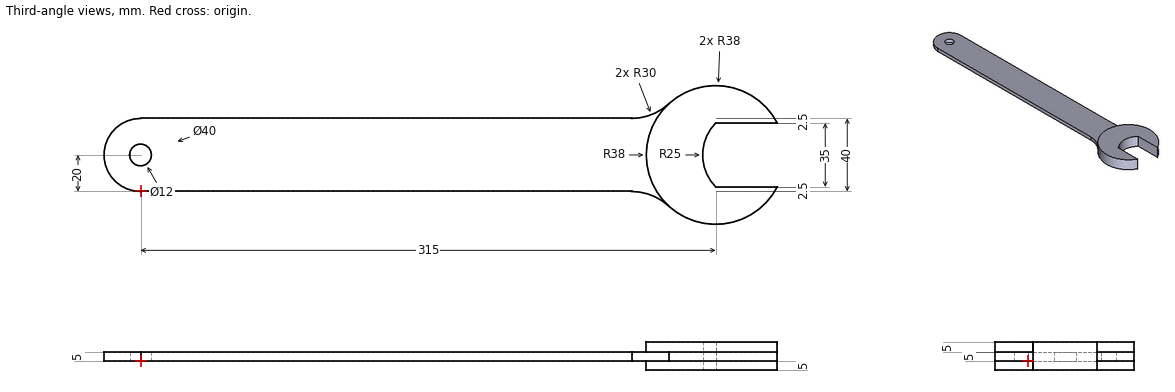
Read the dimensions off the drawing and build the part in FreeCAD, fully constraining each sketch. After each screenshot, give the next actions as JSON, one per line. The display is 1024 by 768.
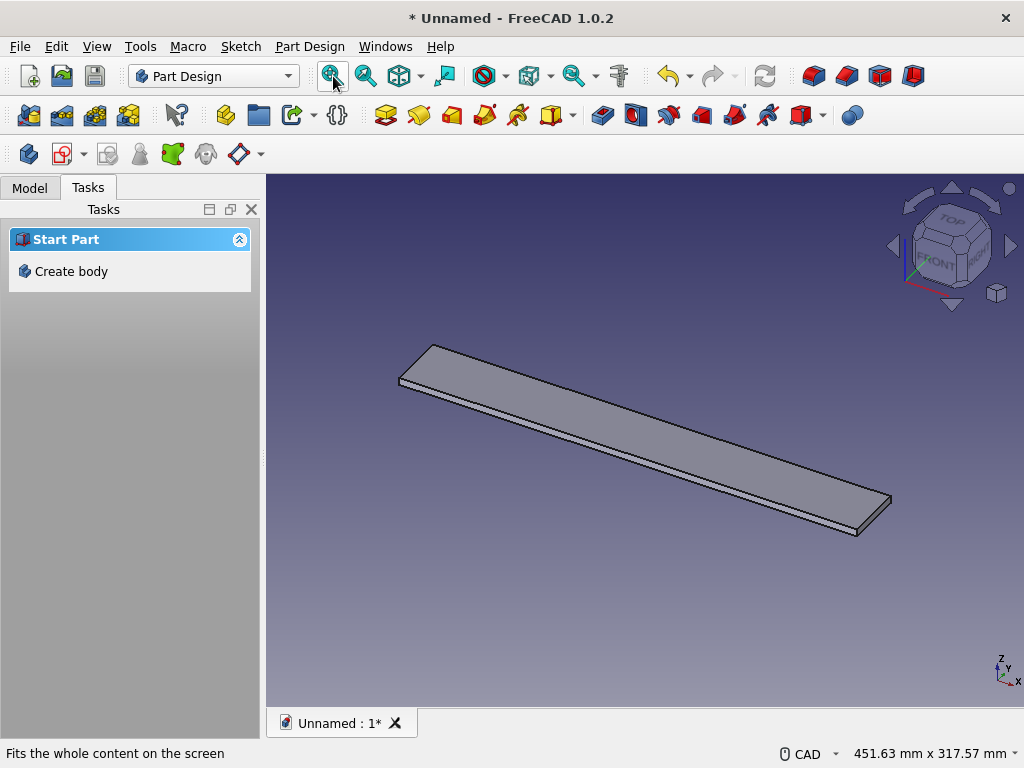
{"action": "left_click", "coordinate": [841, 501]}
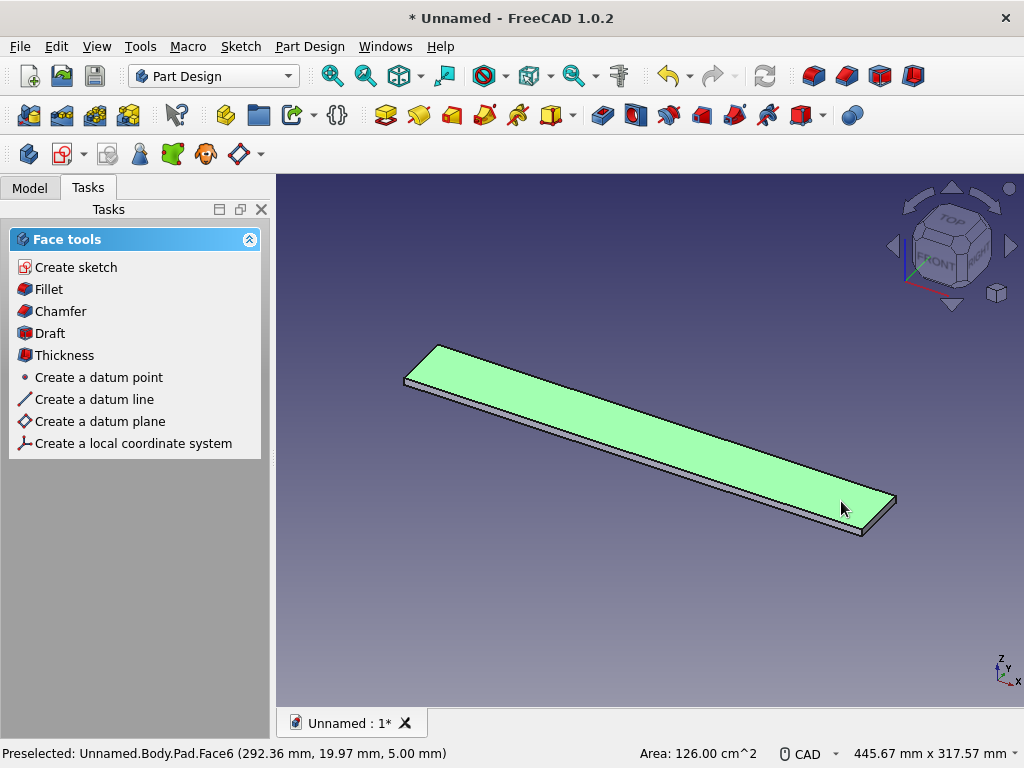
{"action": "left_click", "coordinate": [62, 154]}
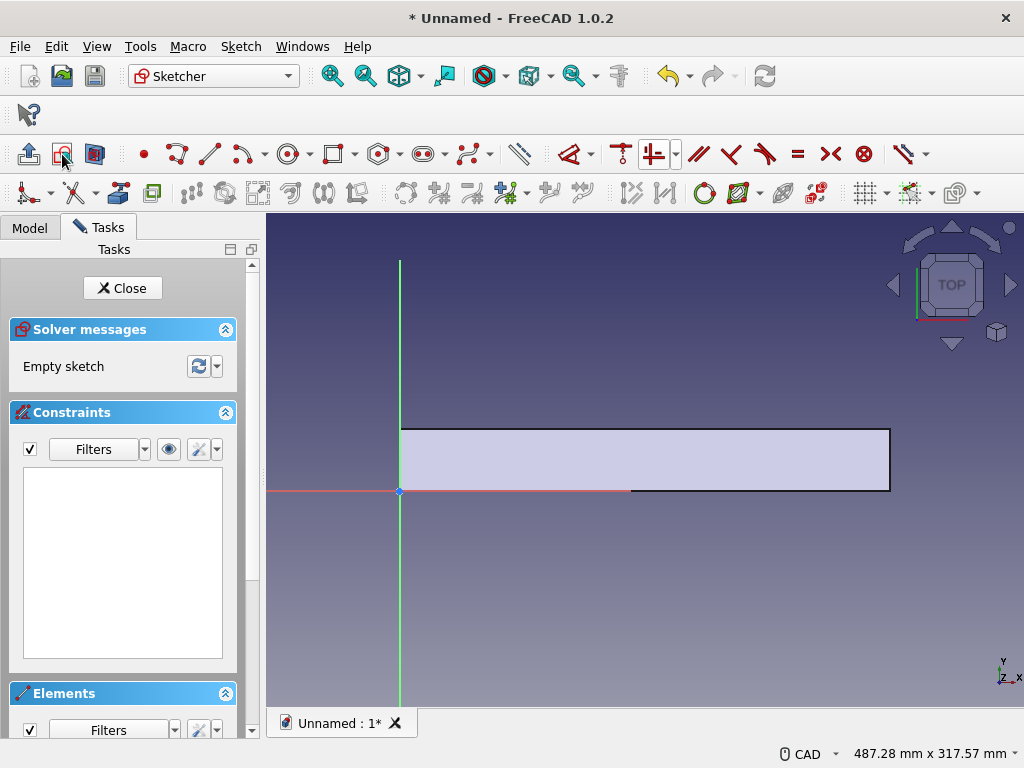
{"action": "scroll", "coordinate": [355, 460], "scroll_direction": "up", "scroll_amount": 8}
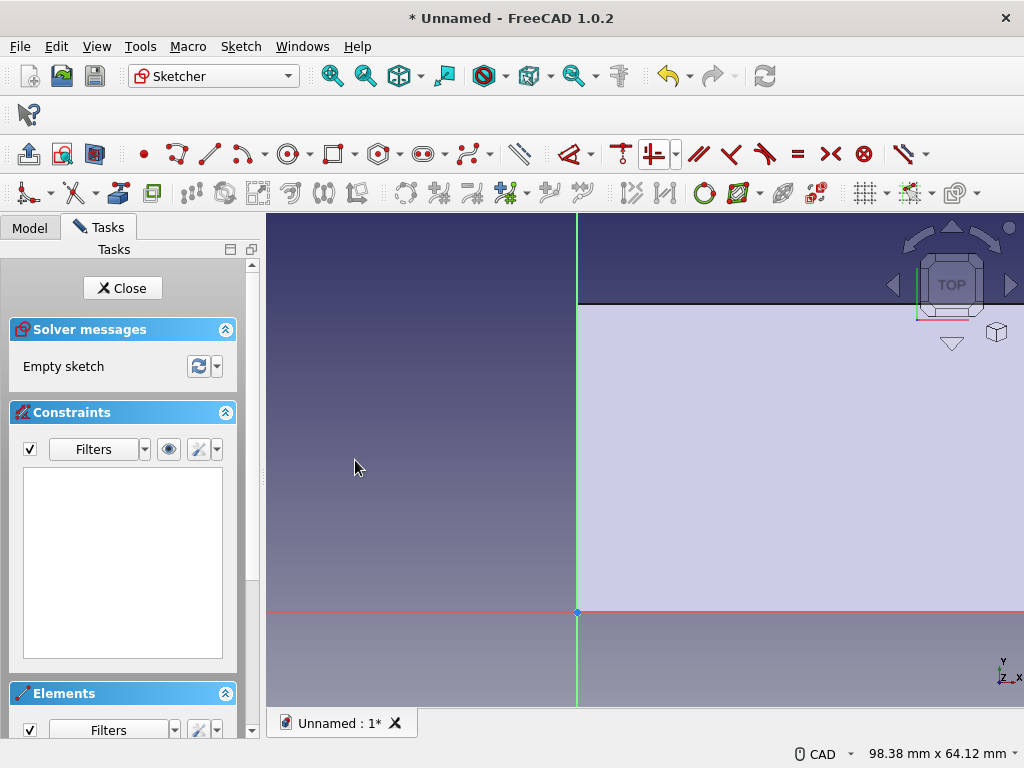
{"action": "left_click", "coordinate": [288, 154]}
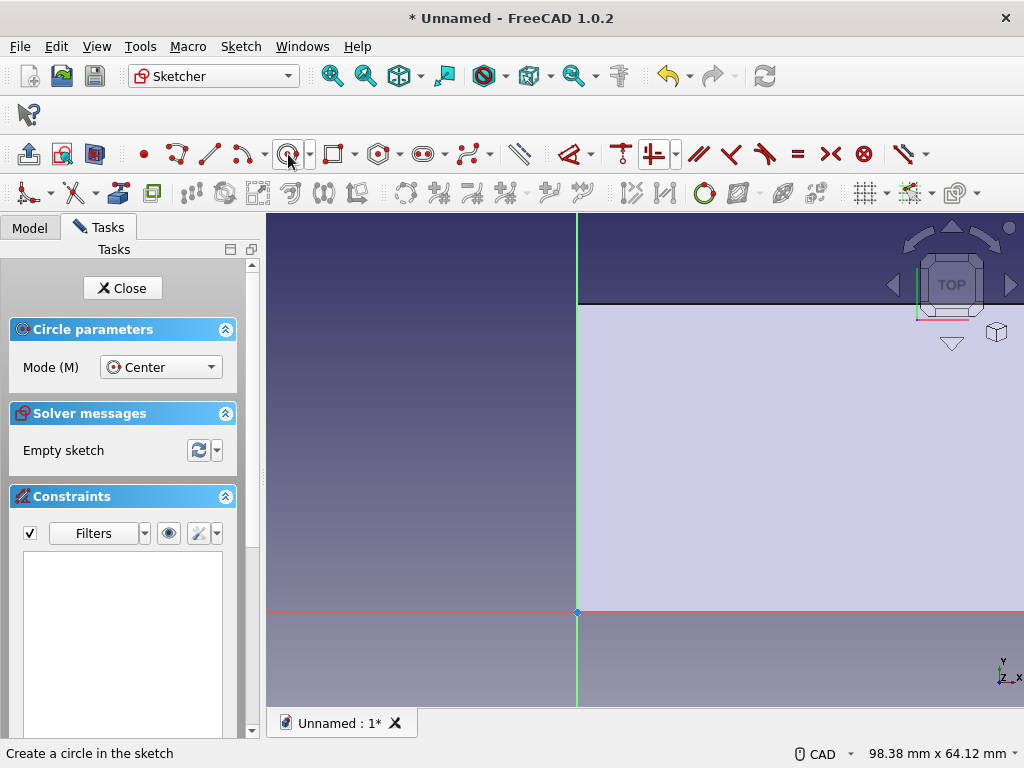
{"action": "left_click", "coordinate": [577, 458]}
{"action": "mouse_move", "coordinate": [686, 349]}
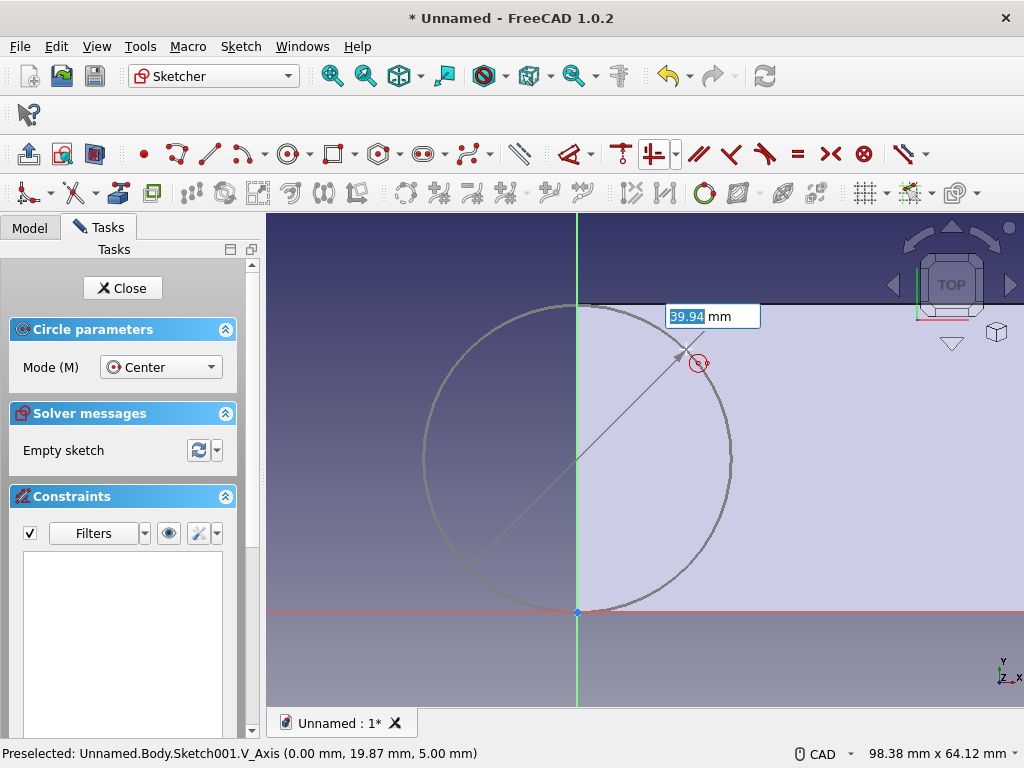
{"action": "type", "text": "40"}
{"action": "key", "text": "Return"}
{"action": "key", "text": "Escape"}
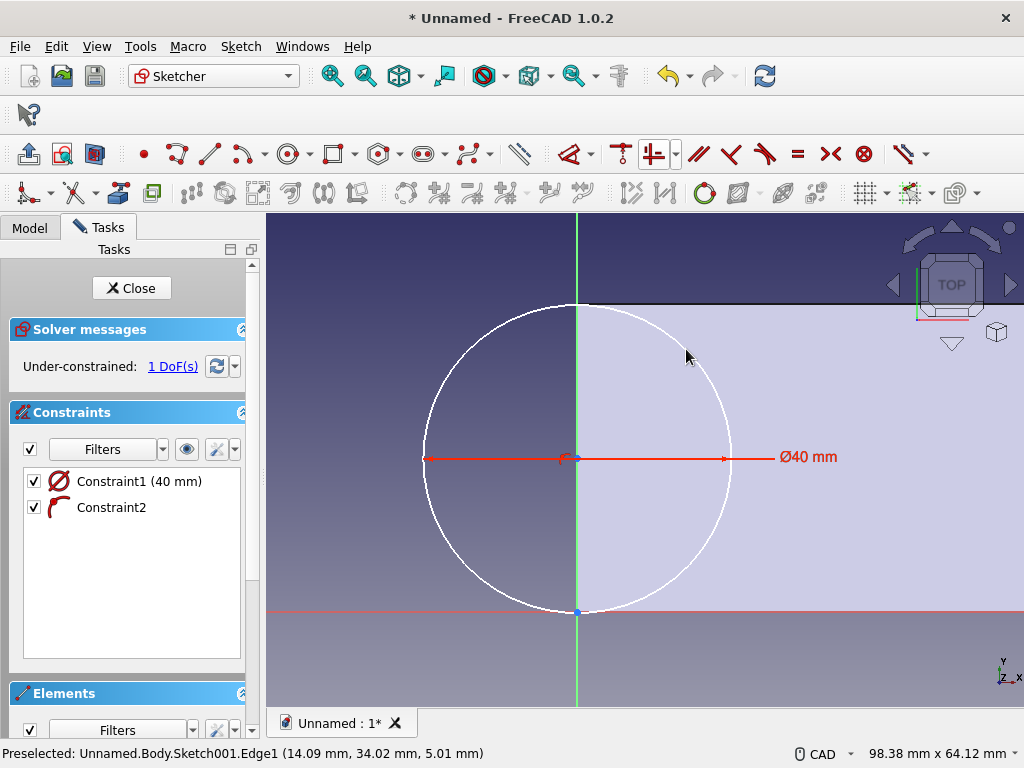
{"action": "left_click", "coordinate": [568, 154]}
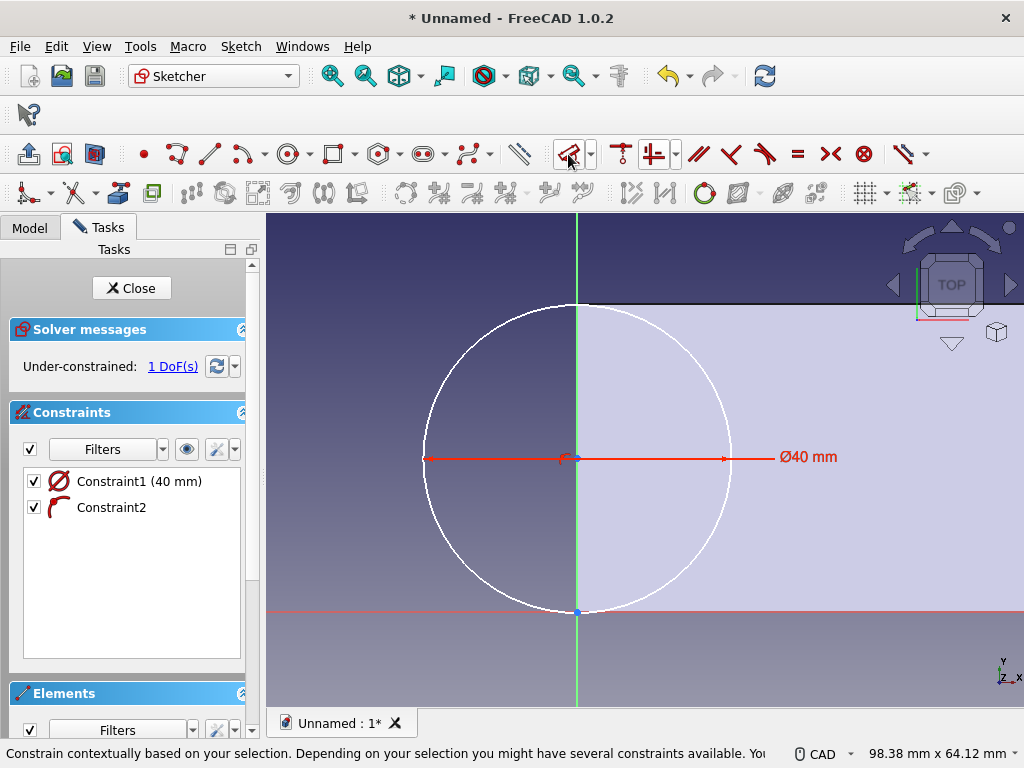
{"action": "left_click", "coordinate": [577, 459]}
{"action": "left_click", "coordinate": [611, 536]}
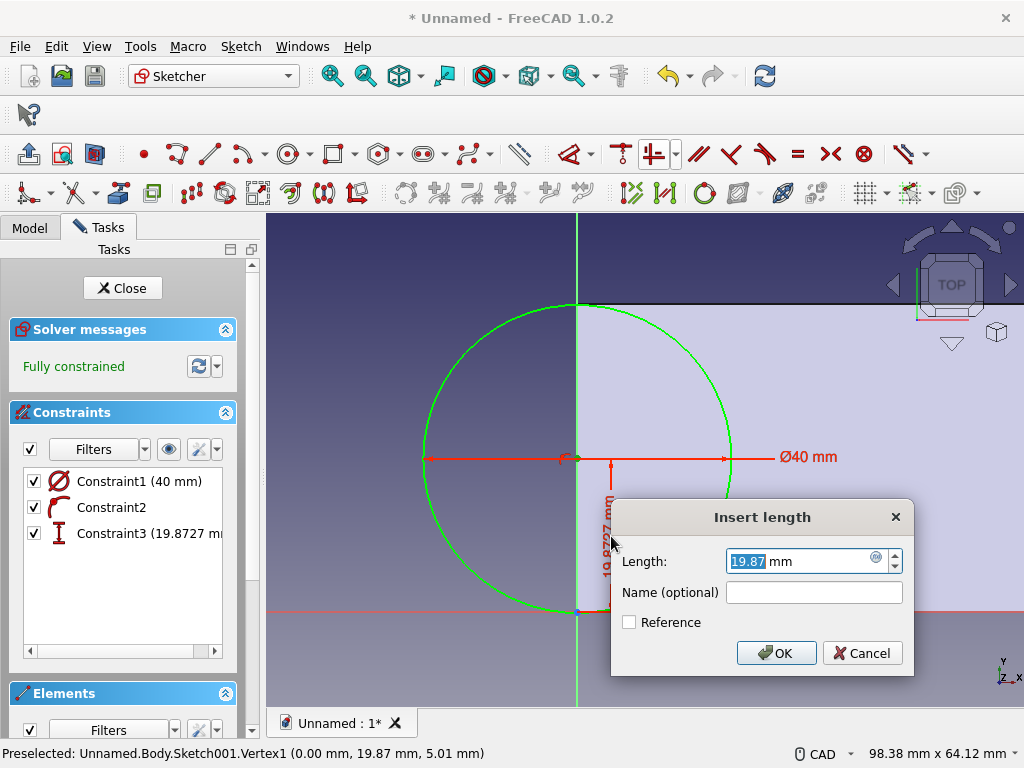
{"action": "type", "text": "20"}
{"action": "key", "text": "Return"}
{"action": "key", "text": "Escape"}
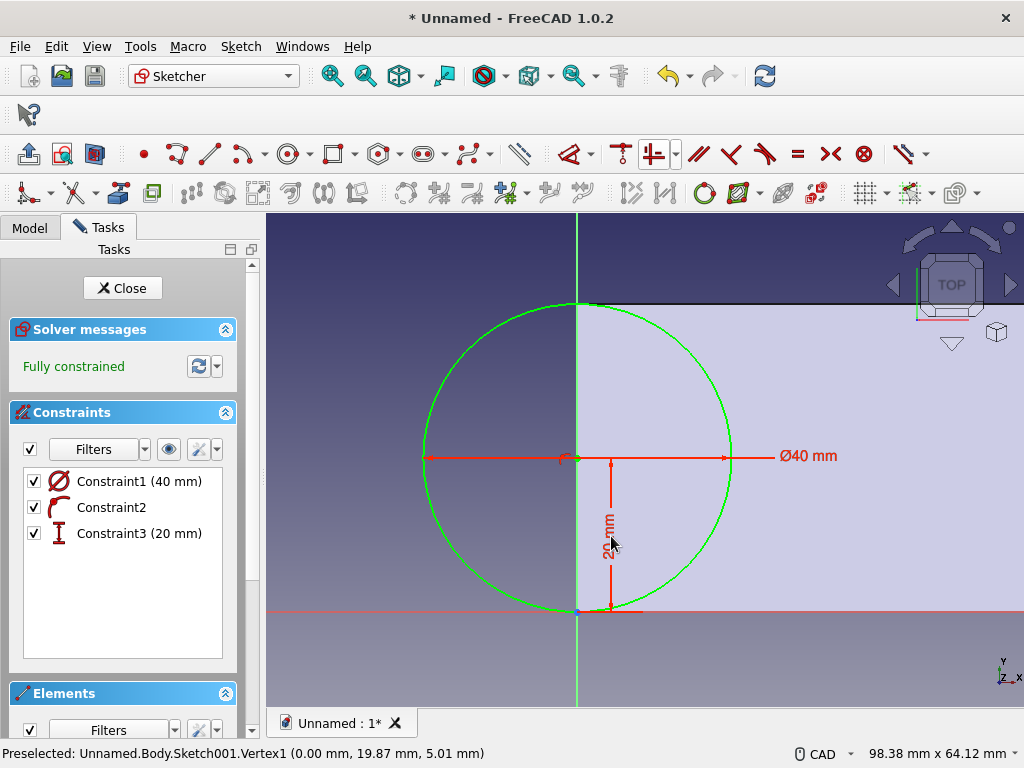
{"action": "left_click", "coordinate": [123, 288]}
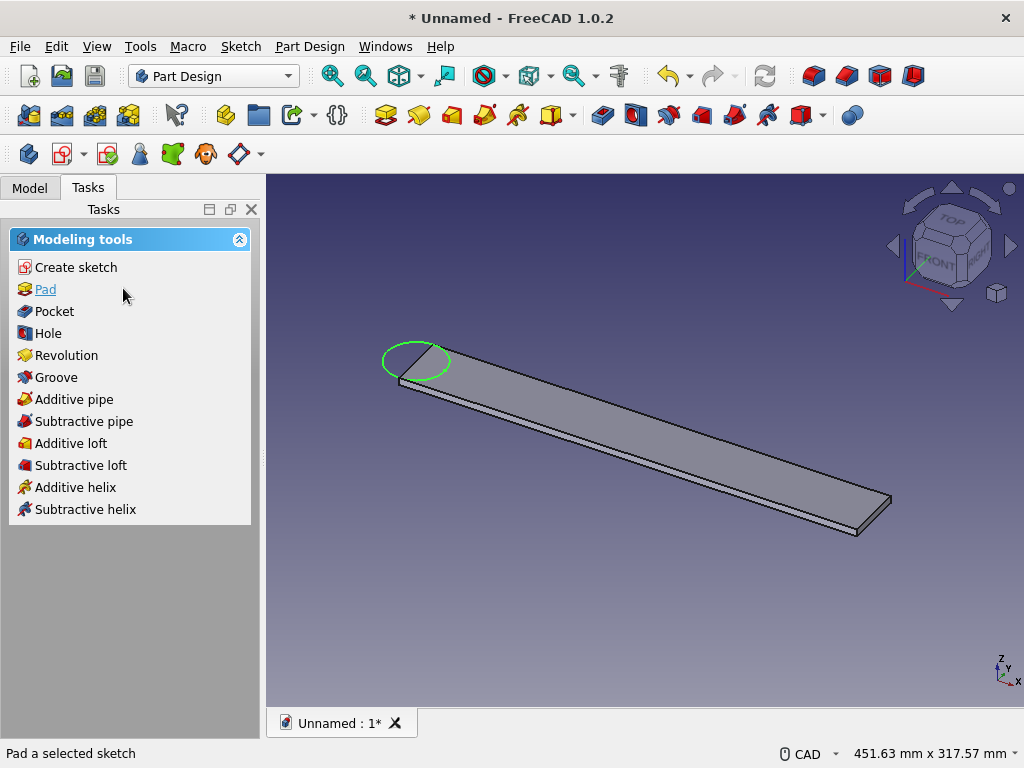
{"action": "left_click", "coordinate": [386, 116]}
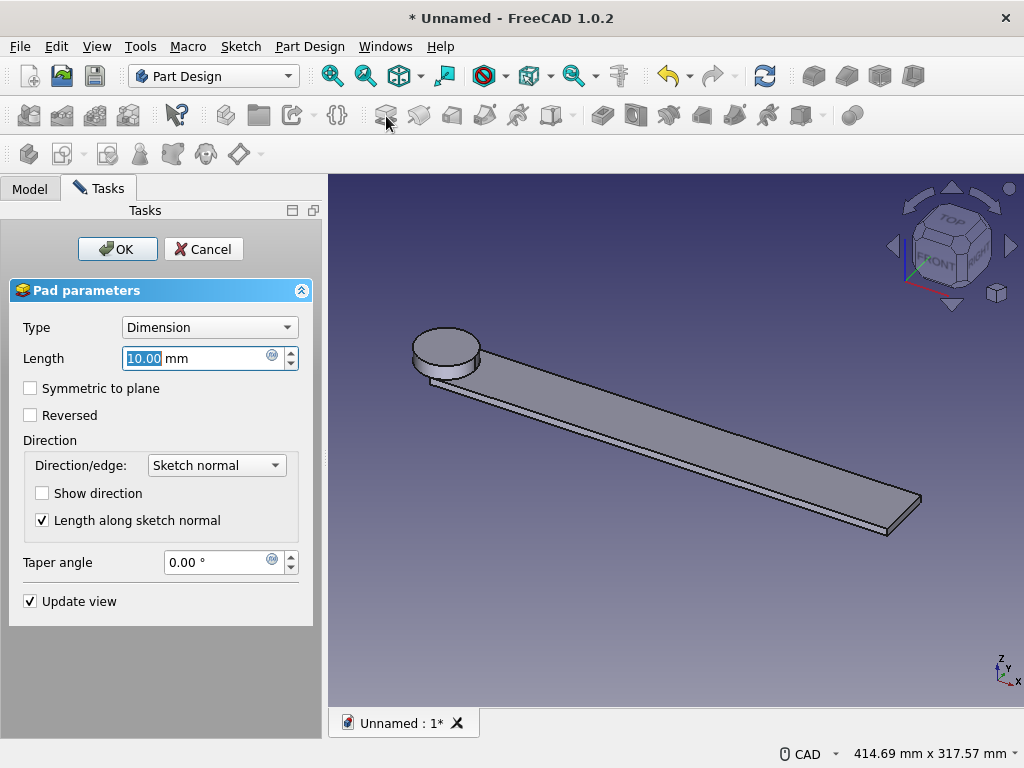
{"action": "type", "text": "5"}
{"action": "key", "text": "Tab"}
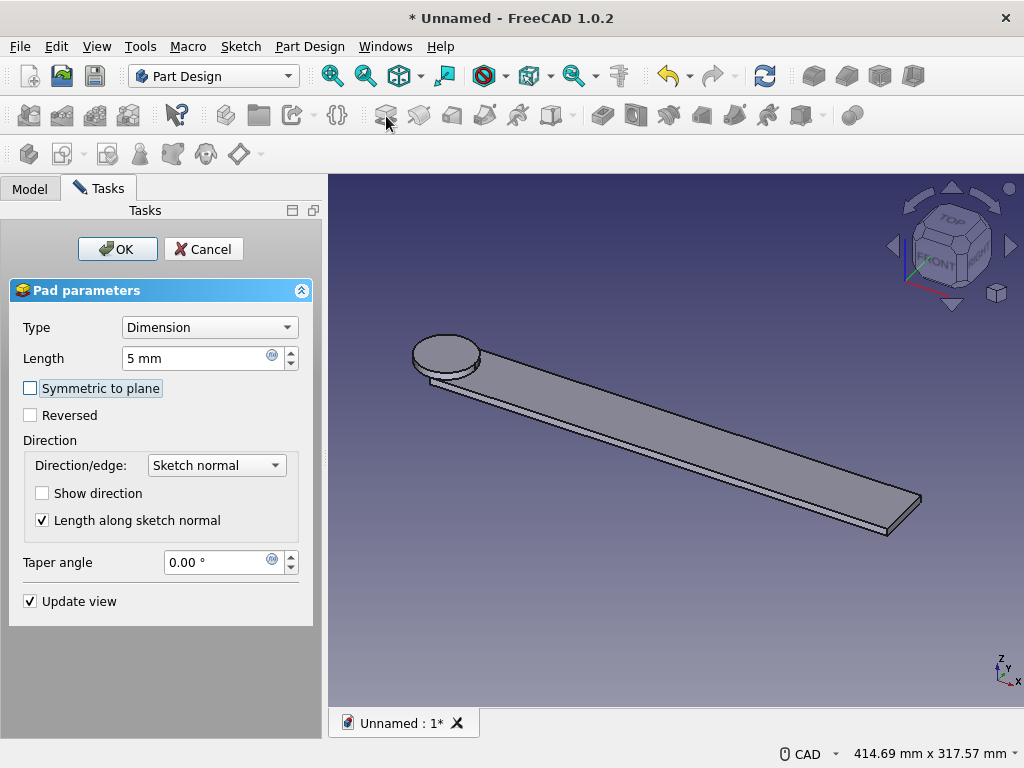
{"action": "left_click", "coordinate": [31, 415]}